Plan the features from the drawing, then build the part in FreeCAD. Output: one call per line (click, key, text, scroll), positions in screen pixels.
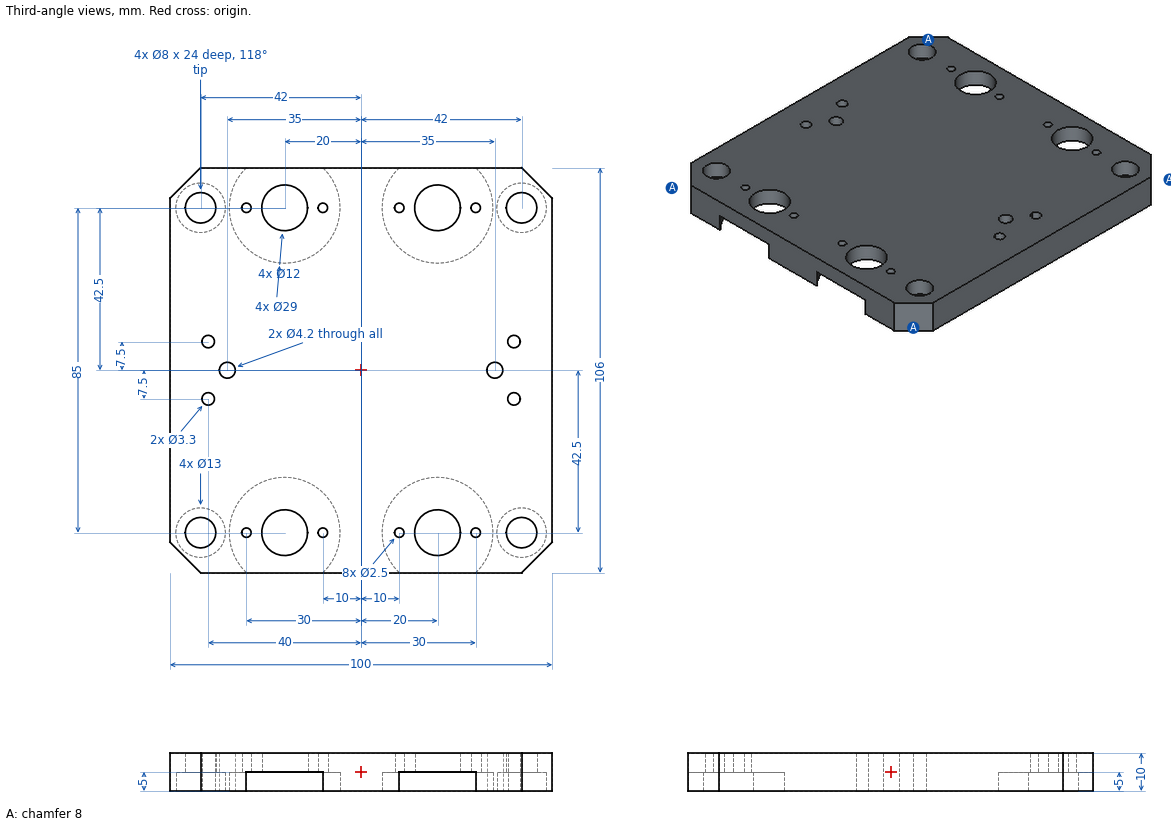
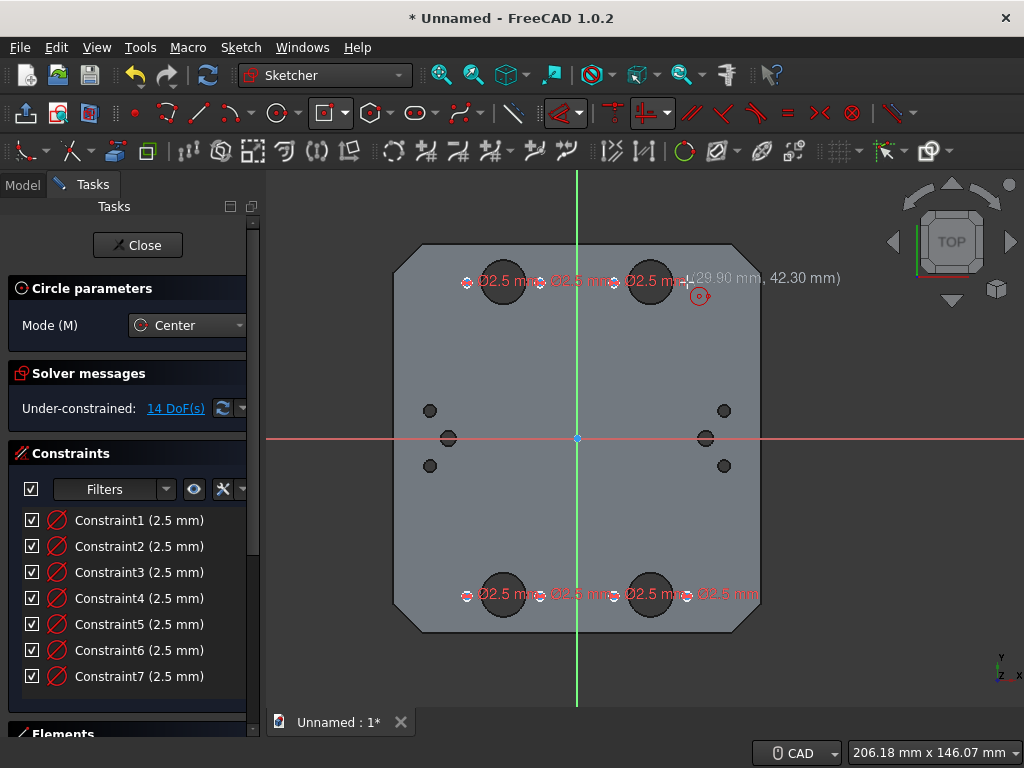
click(687, 282)
move(691, 279)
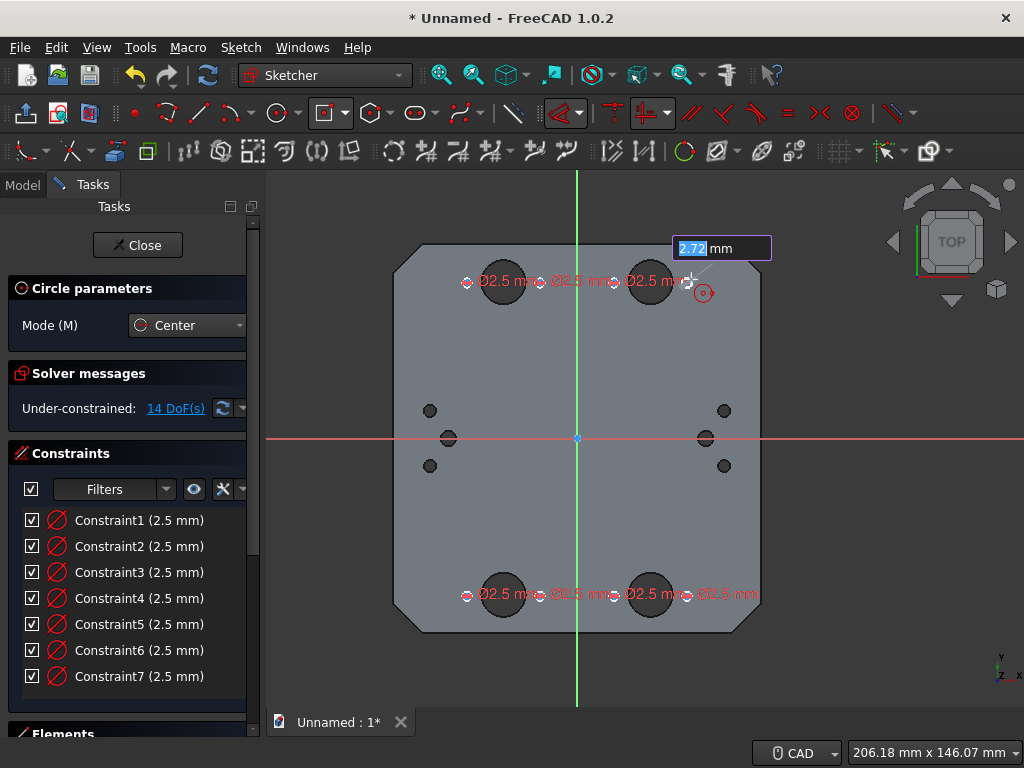
text(2.5)
key(Return)
key(Escape)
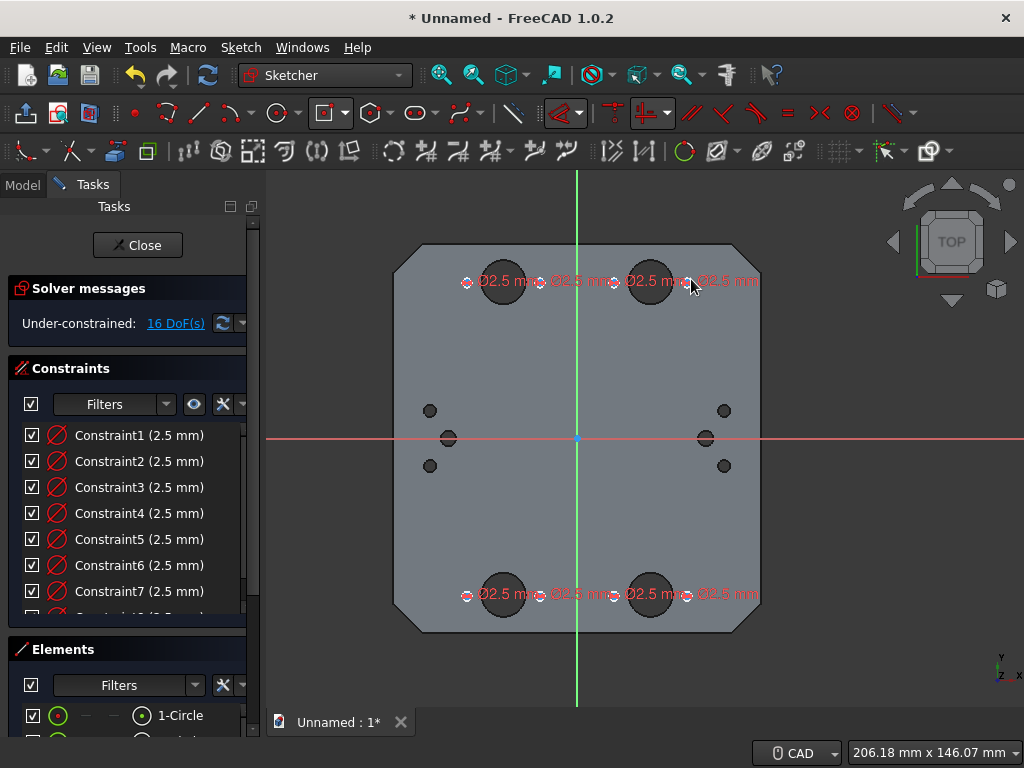
click(614, 596)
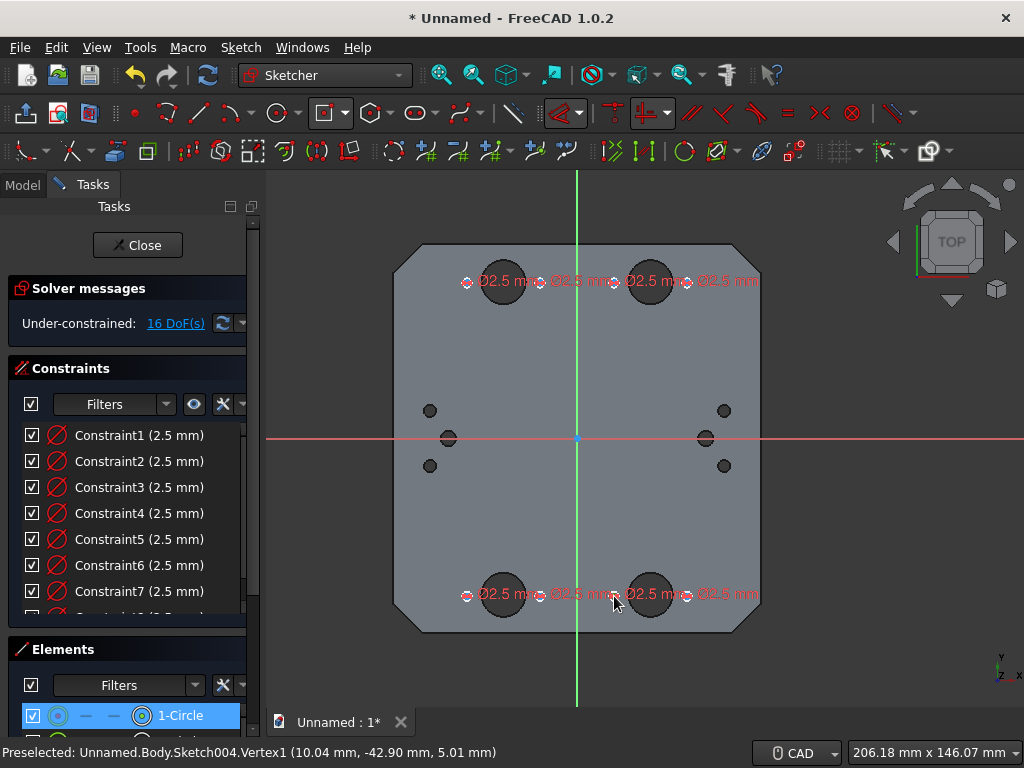
click(687, 596)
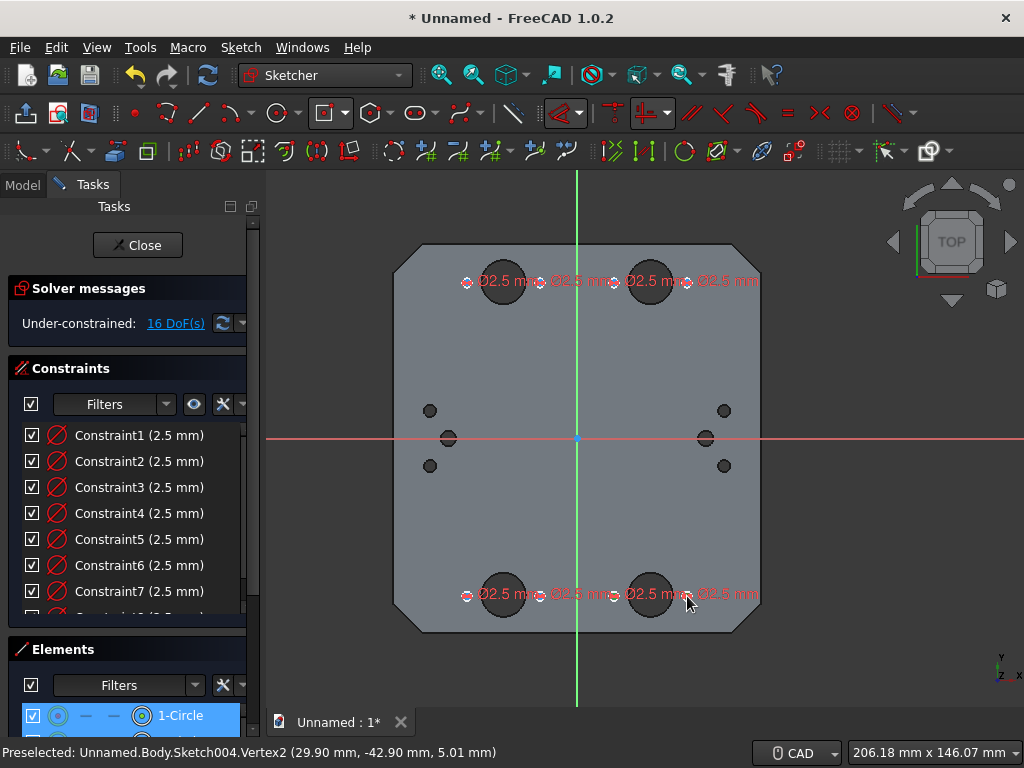
key(h)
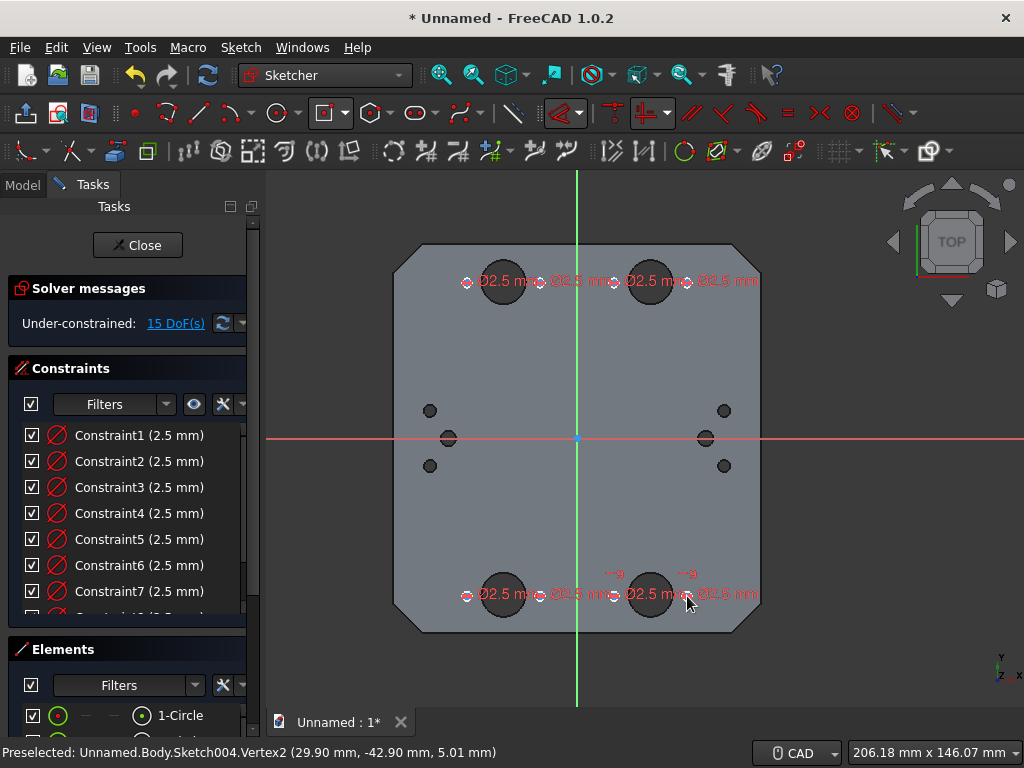
click(614, 596)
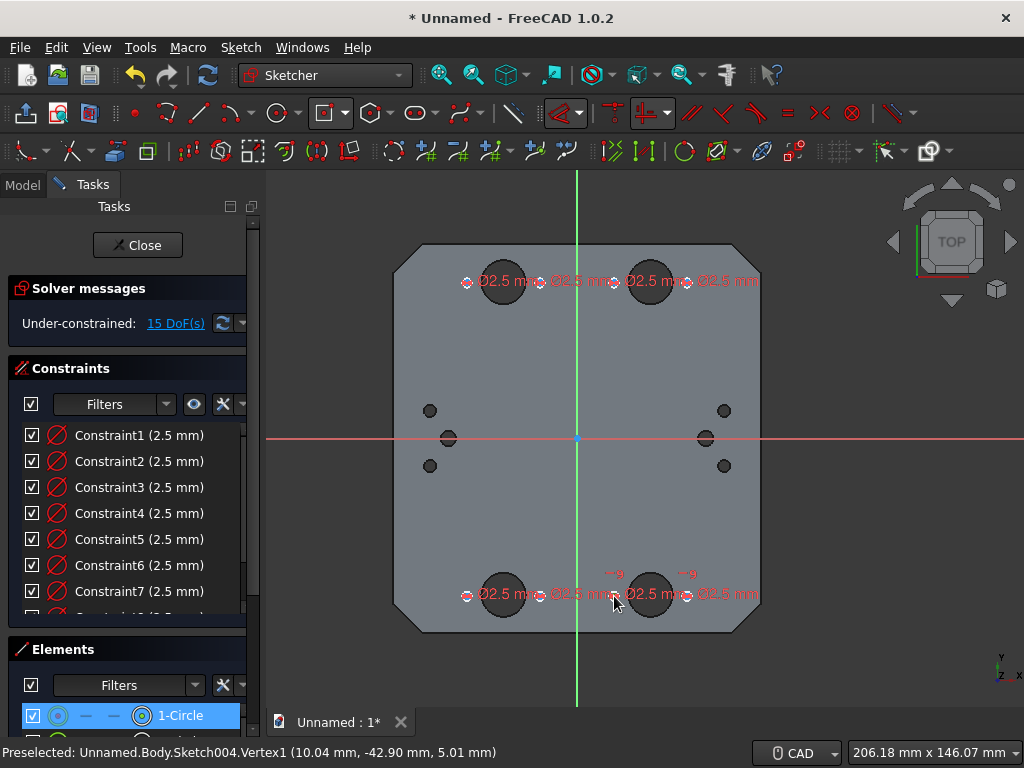
click(540, 596)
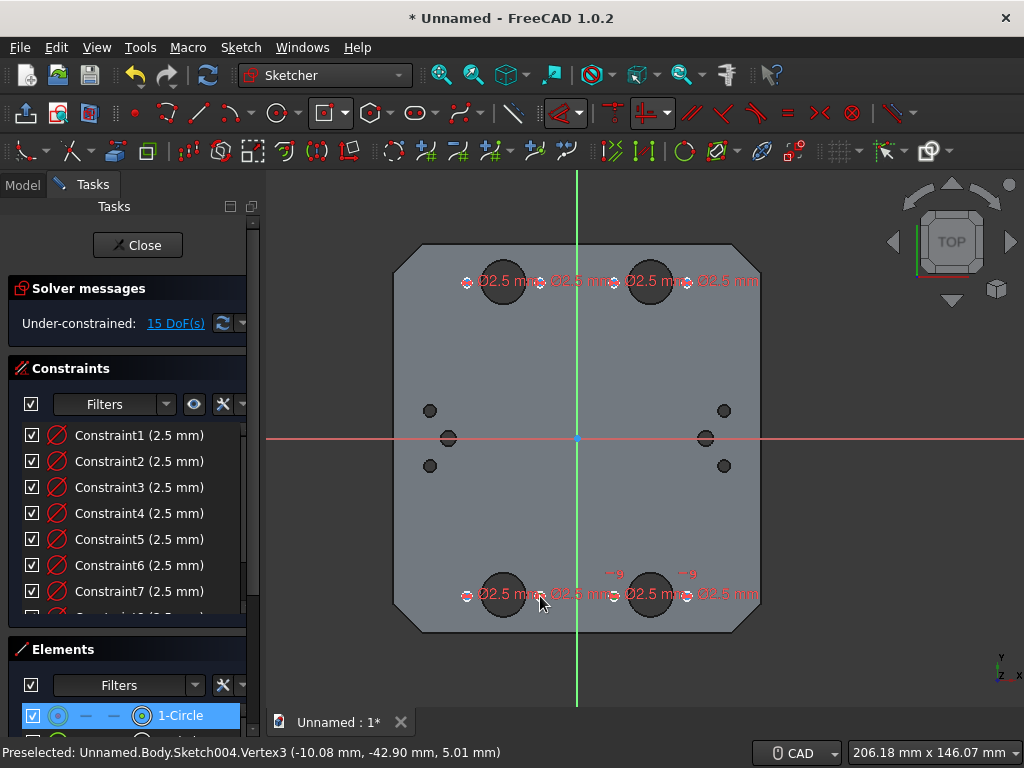
click(670, 114)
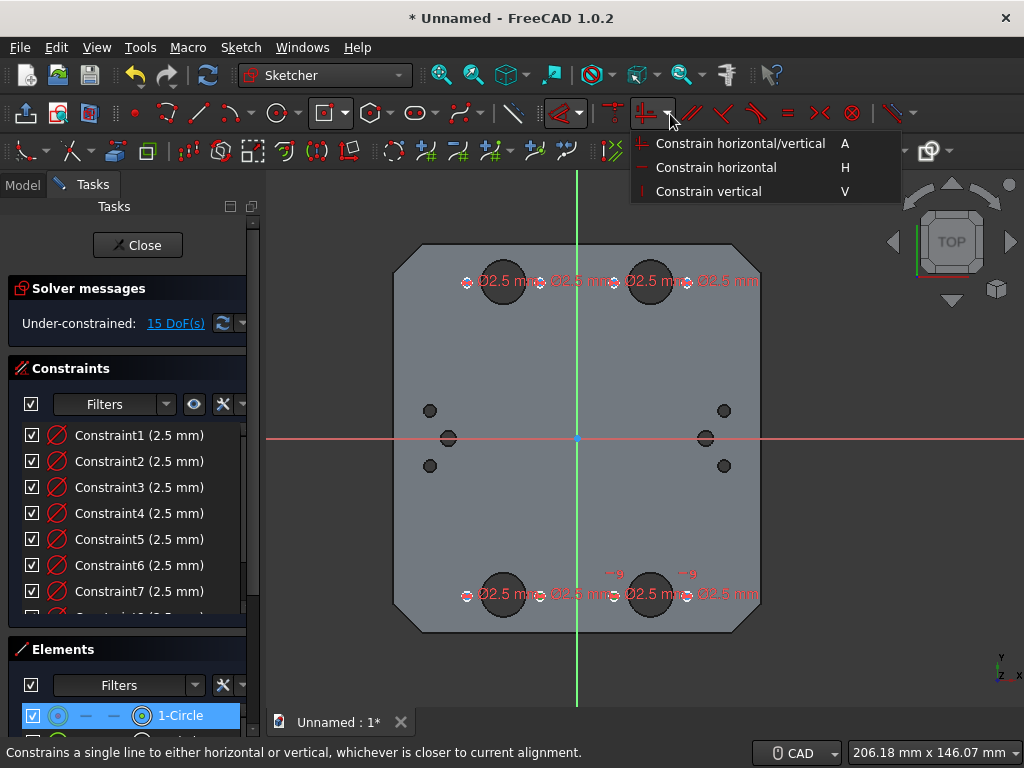
click(766, 167)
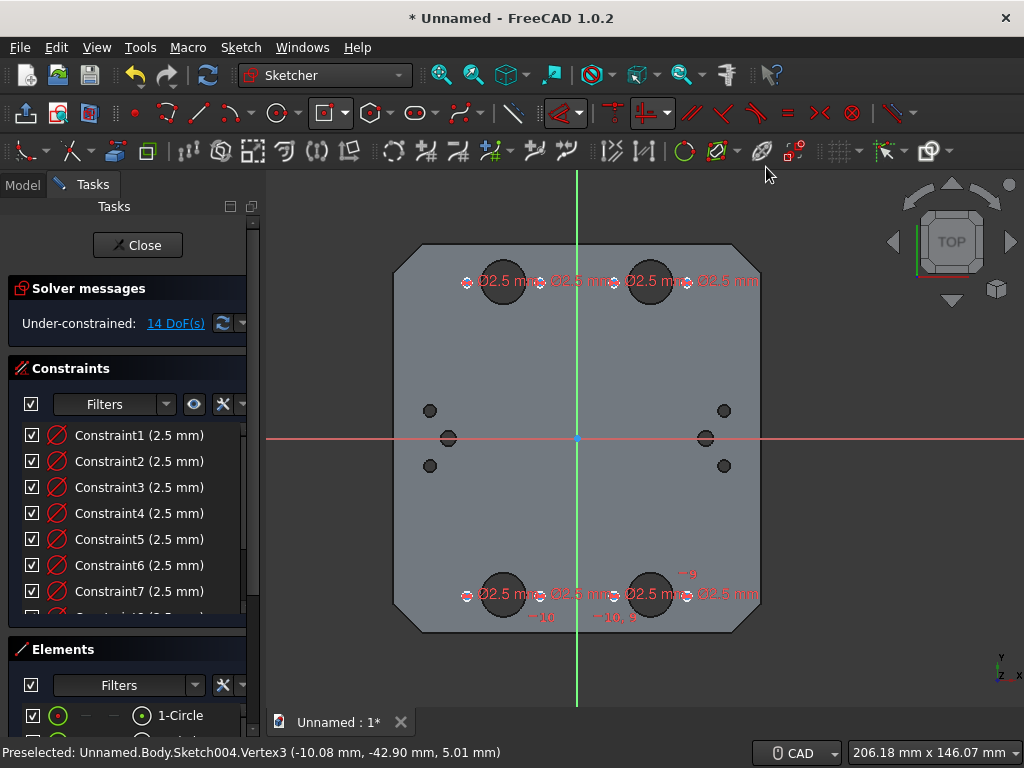
click(540, 596)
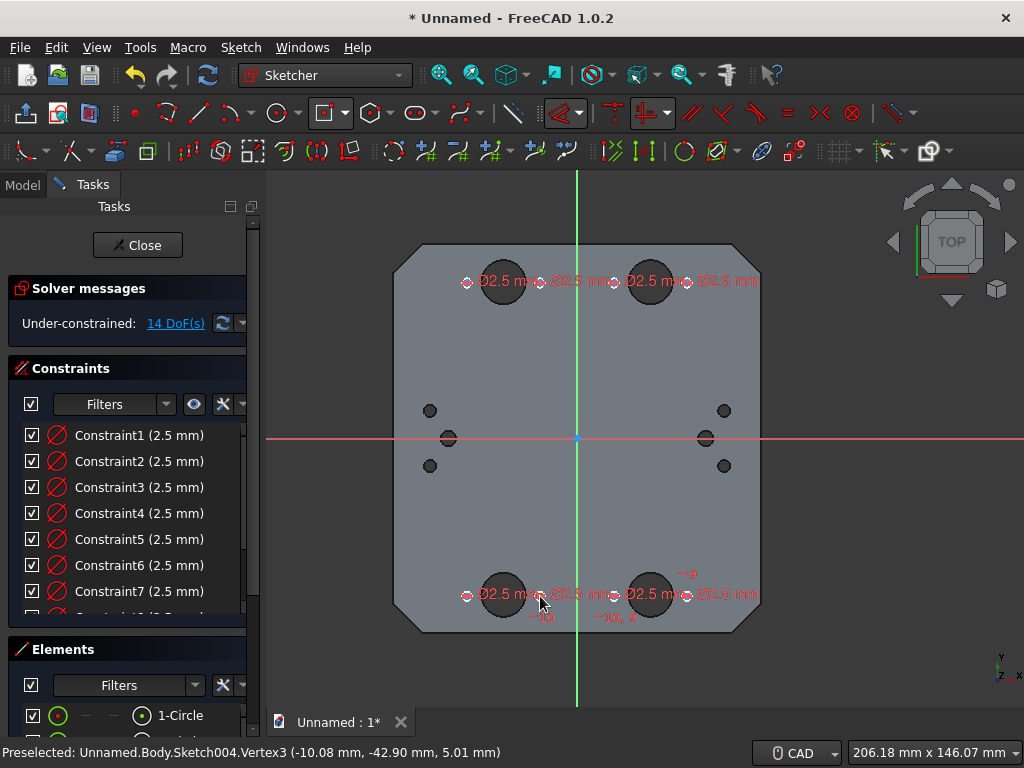
click(467, 596)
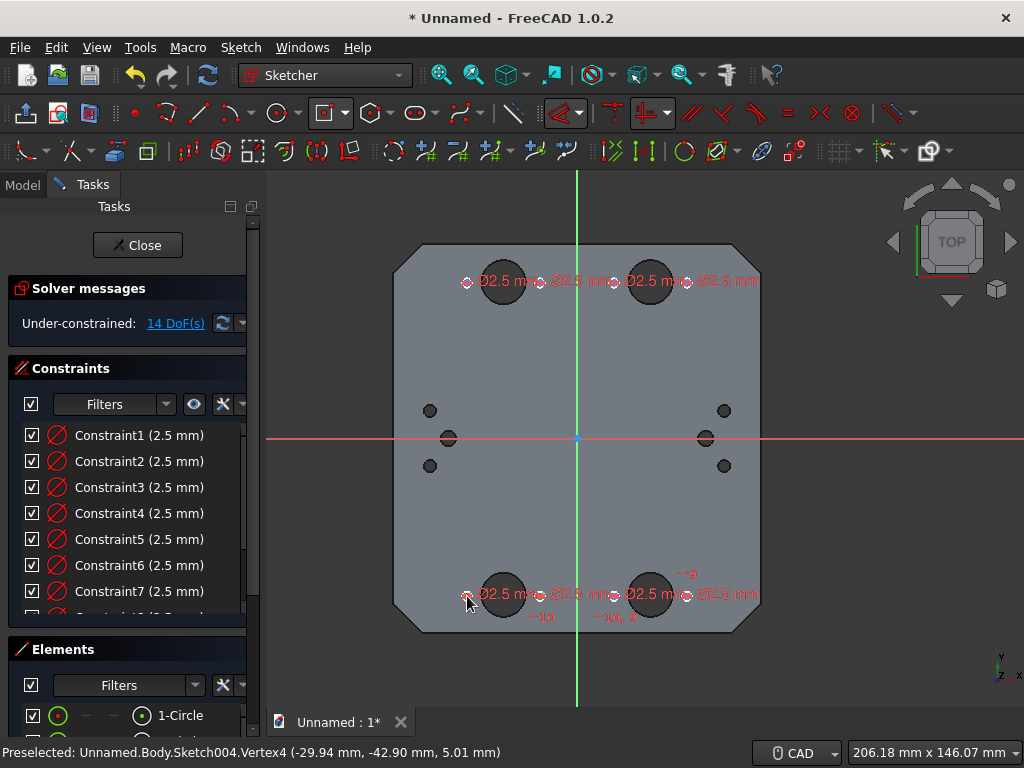
key(h)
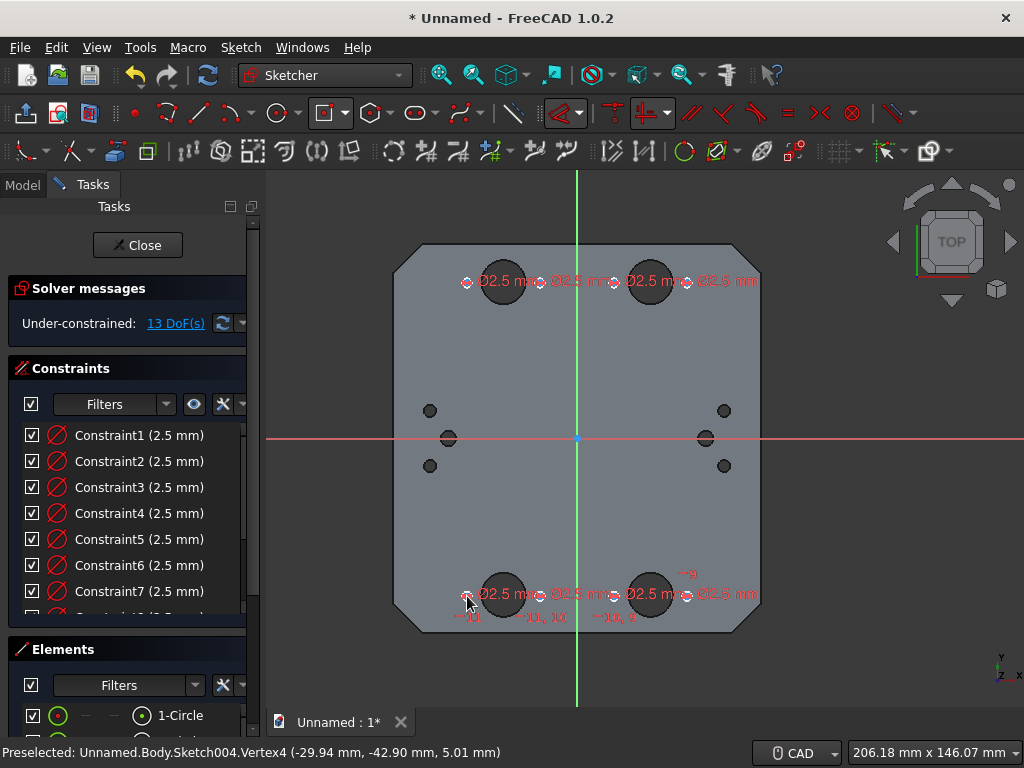
click(540, 596)